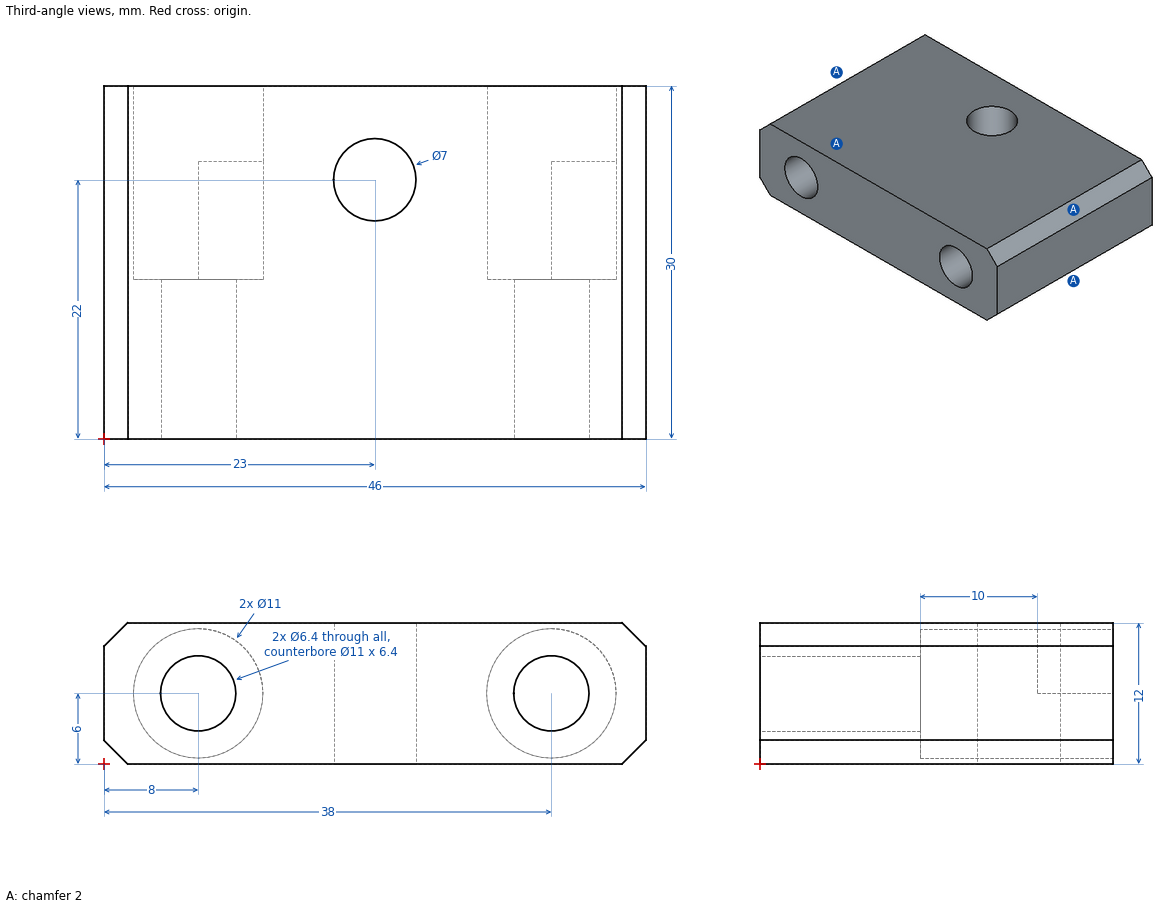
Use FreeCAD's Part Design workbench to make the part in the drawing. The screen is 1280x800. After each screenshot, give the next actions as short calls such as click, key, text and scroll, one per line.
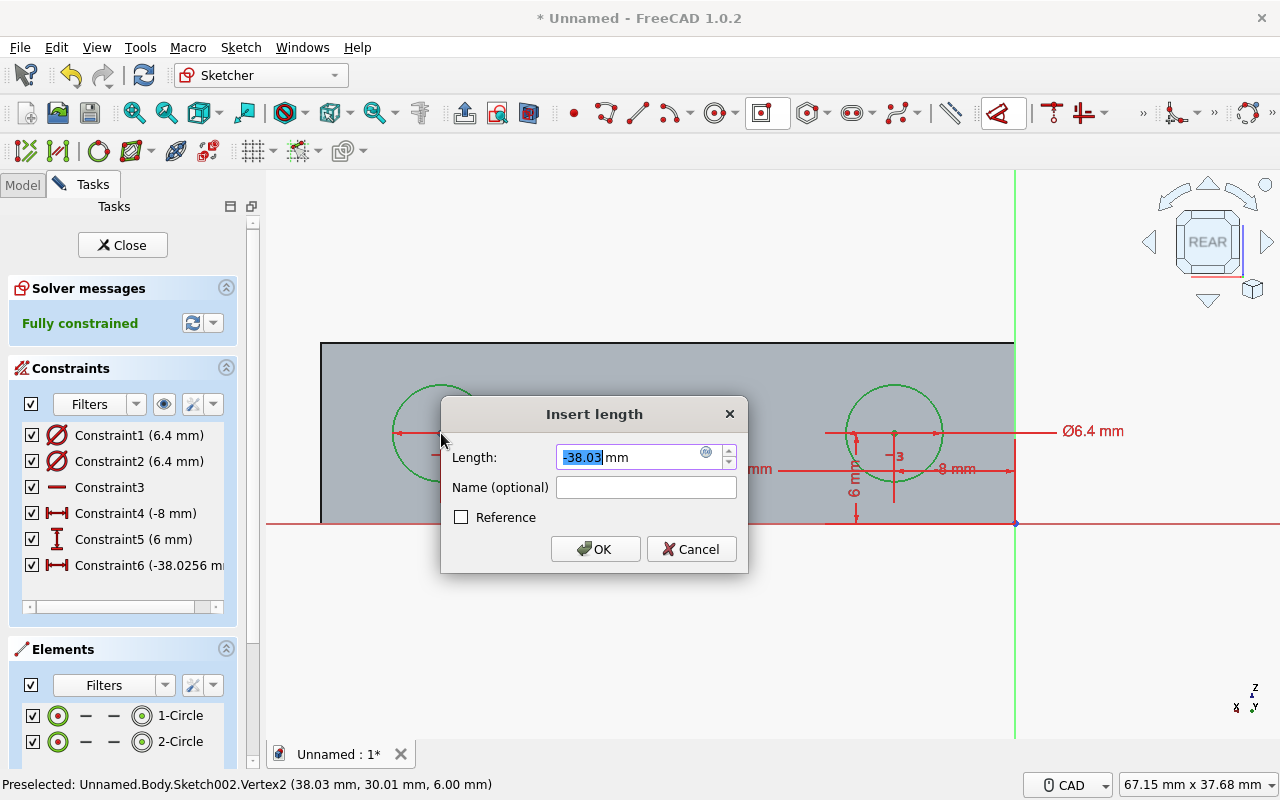
text(-38)
key(Return)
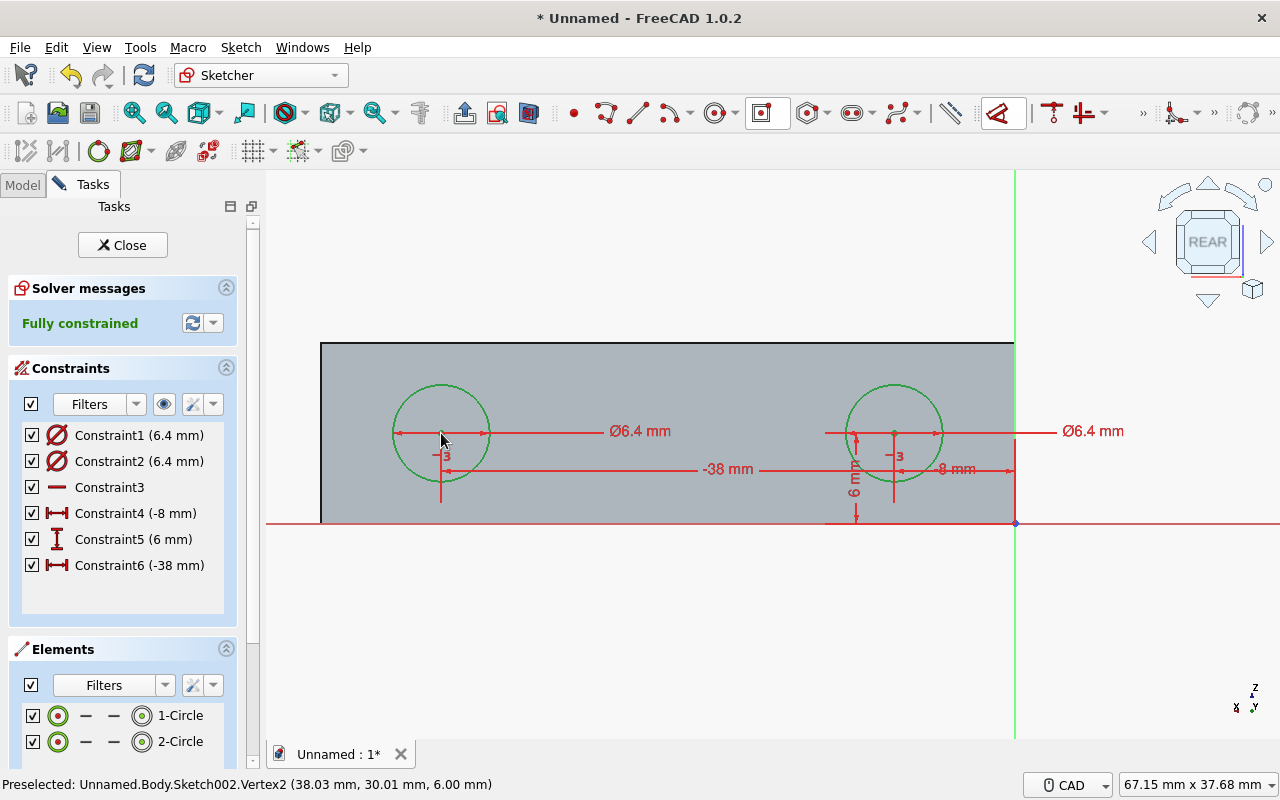
click(123, 245)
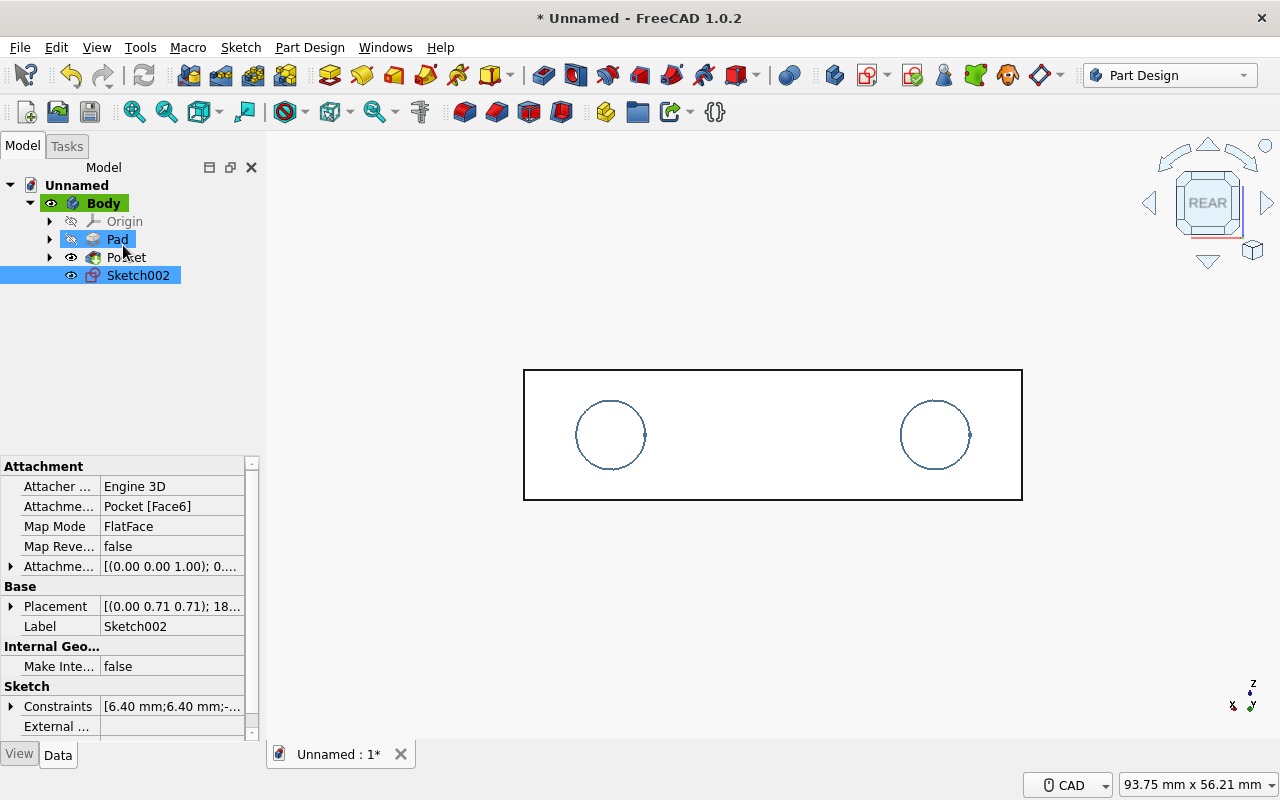
click(576, 76)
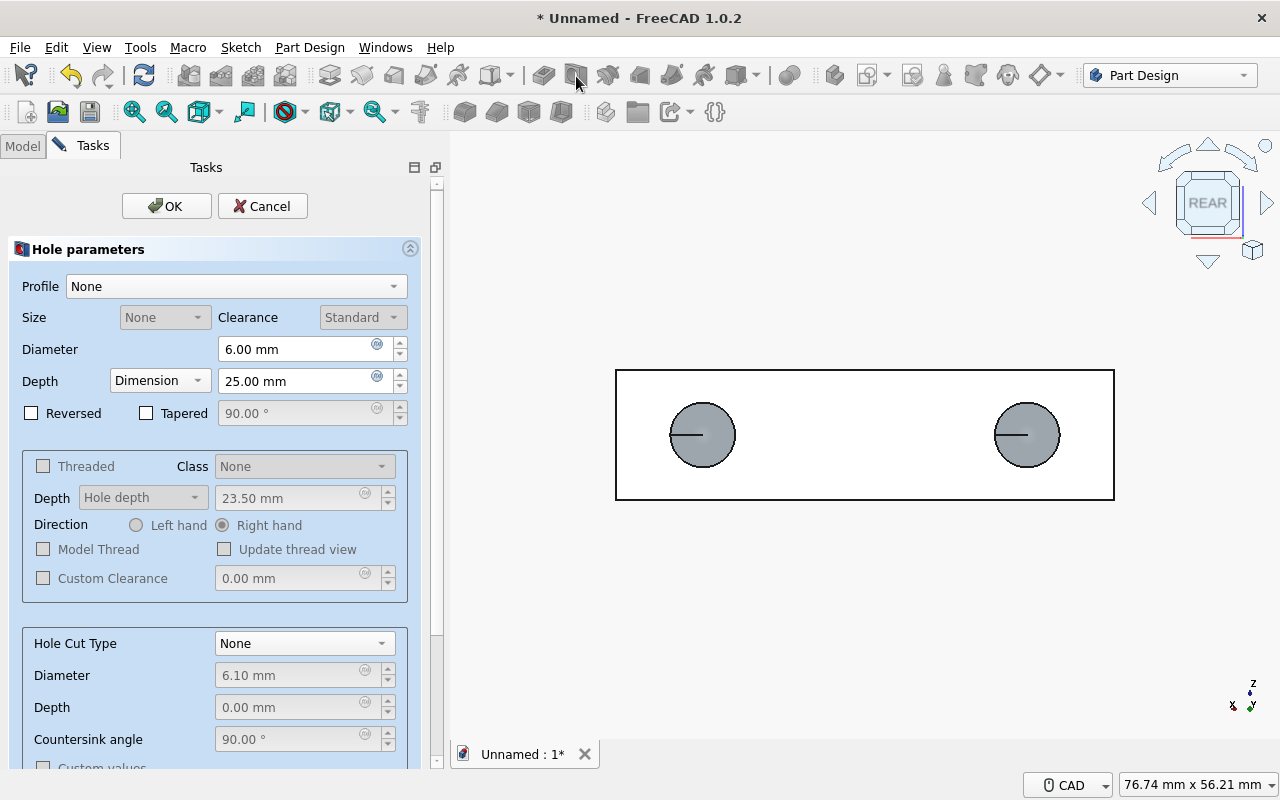
triple_click(305, 349)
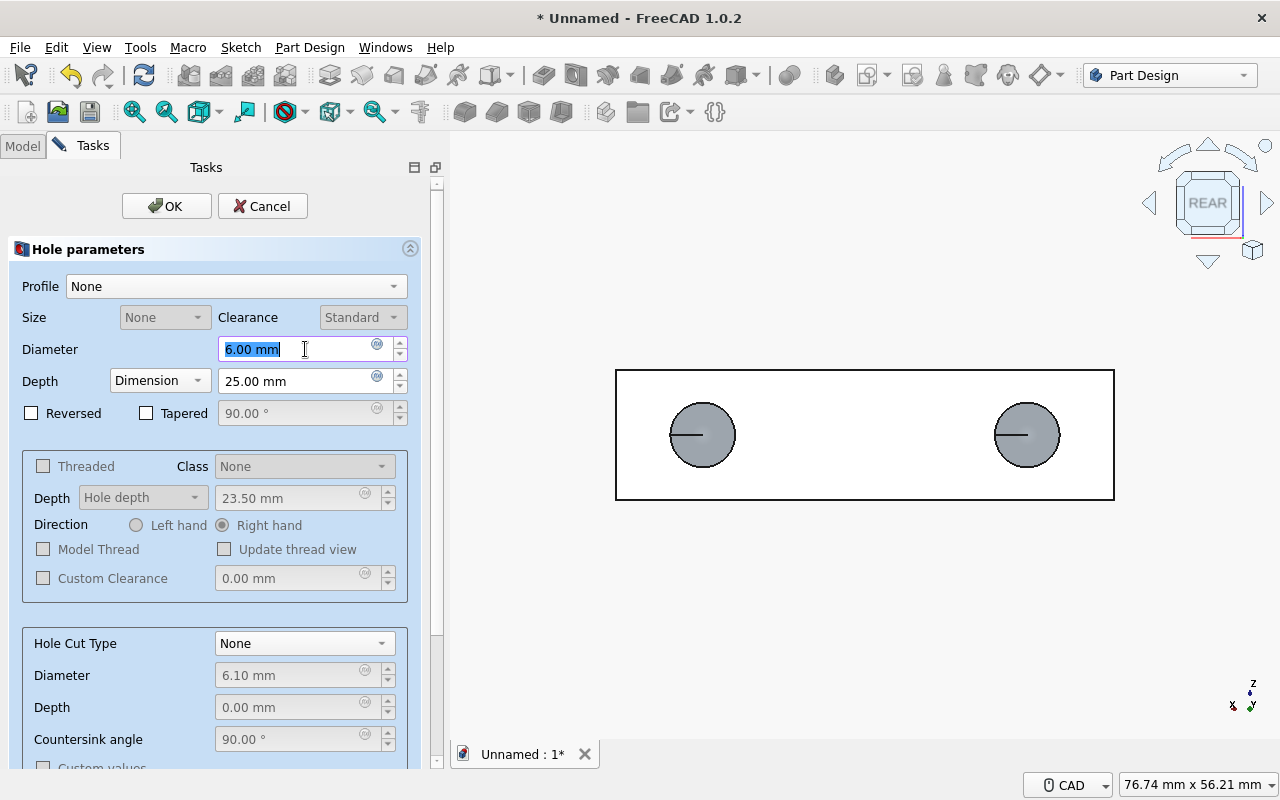
text(6.4)
key(Tab)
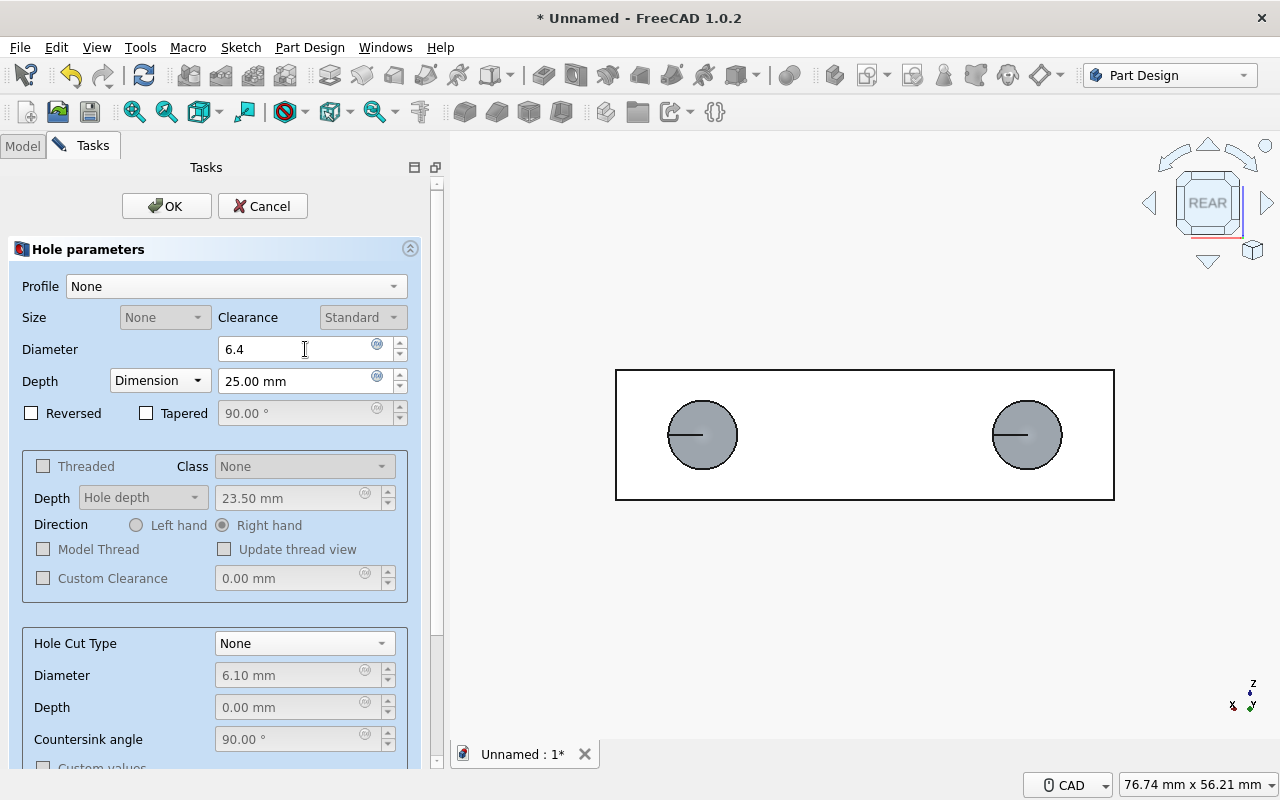
click(161, 380)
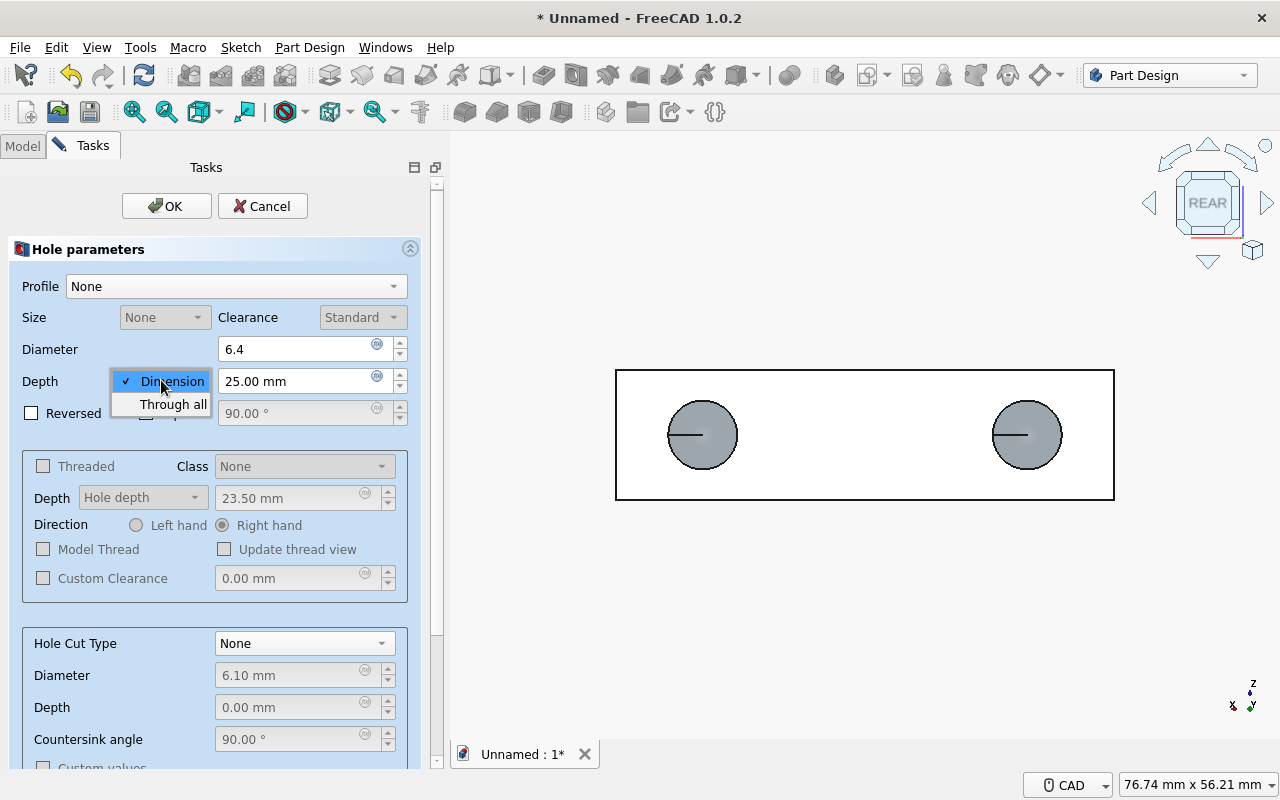
click(160, 404)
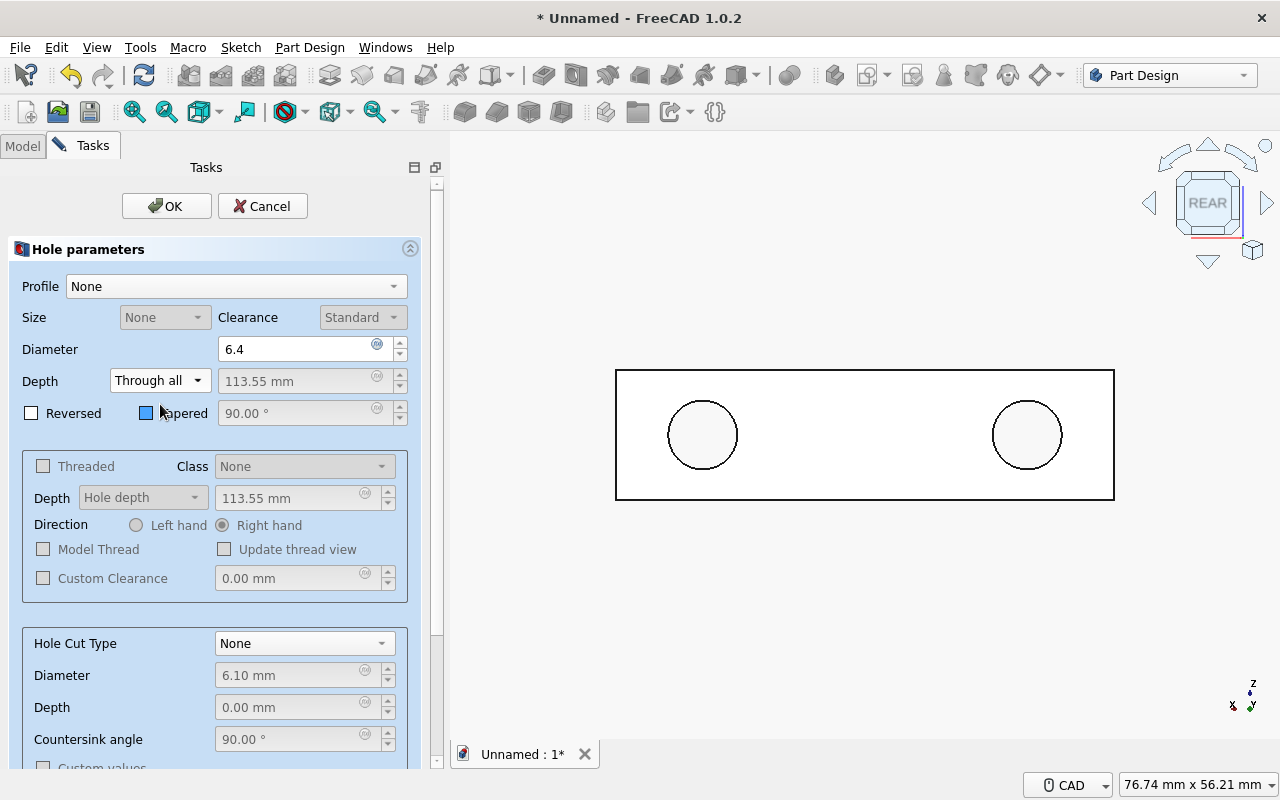
click(306, 644)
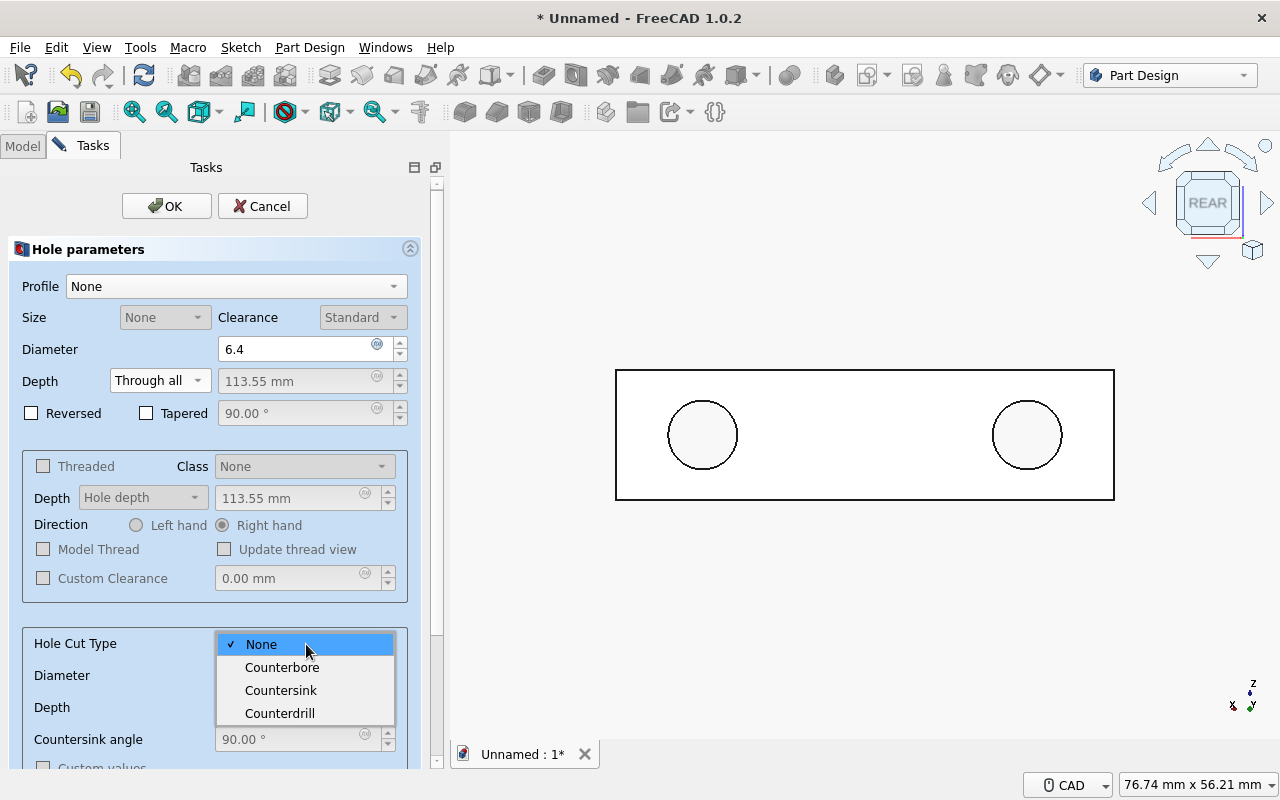
click(304, 668)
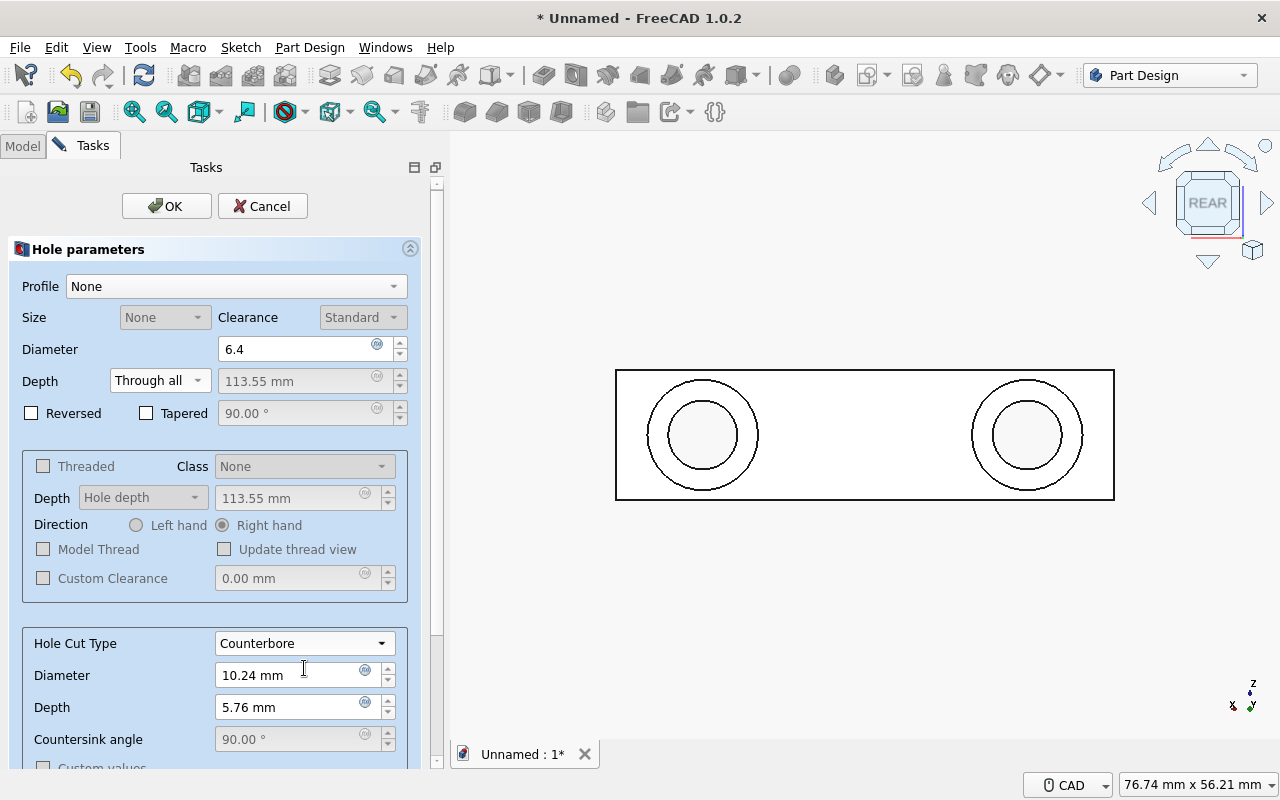
triple_click(298, 675)